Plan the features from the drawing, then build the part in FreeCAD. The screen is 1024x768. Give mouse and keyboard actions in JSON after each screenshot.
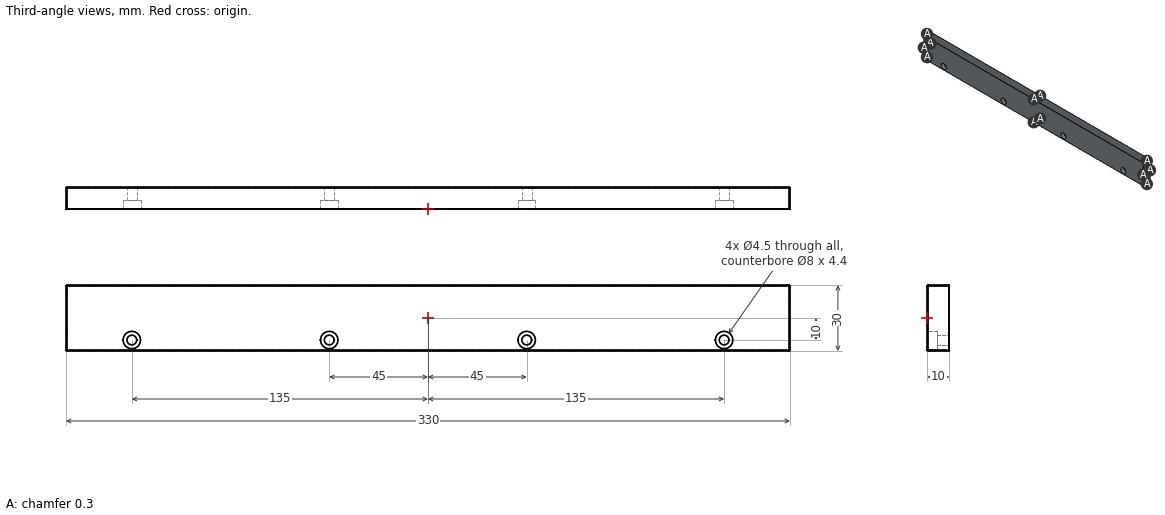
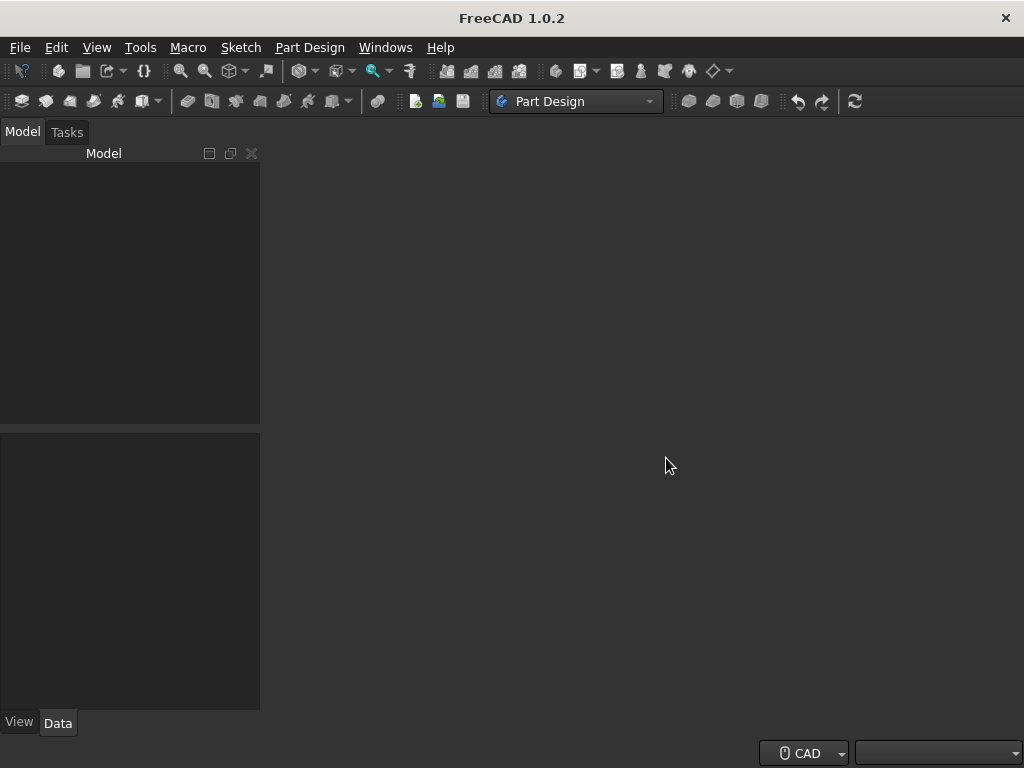
{"action": "left_click", "coordinate": [416, 102]}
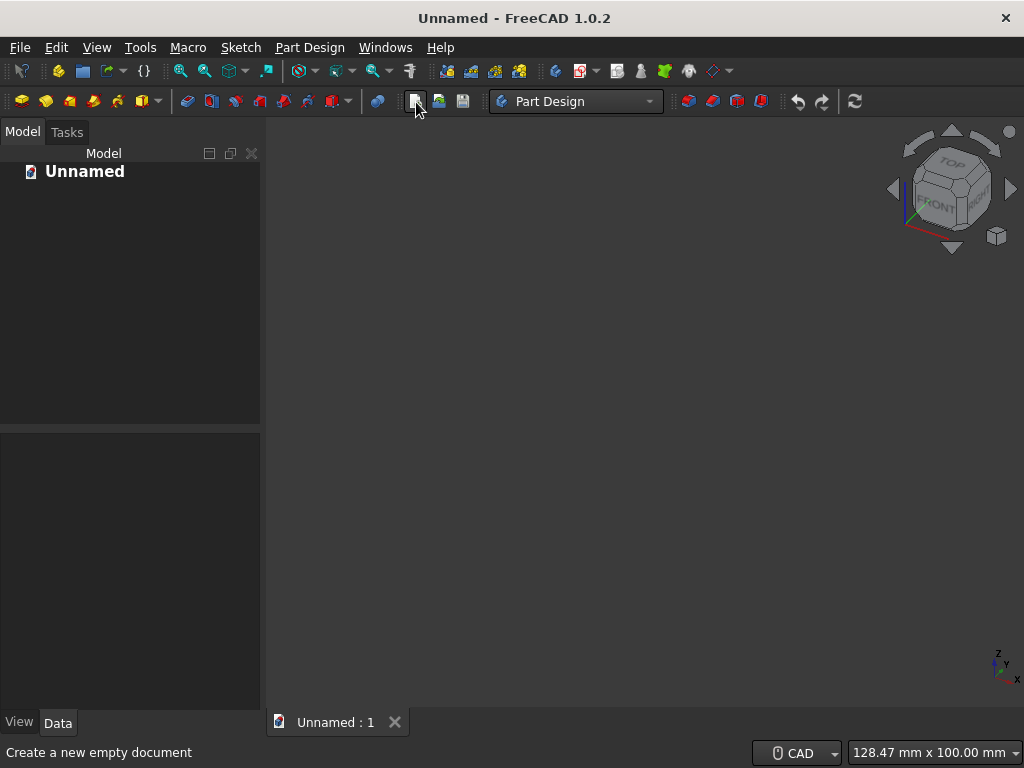
{"action": "left_click", "coordinate": [580, 72]}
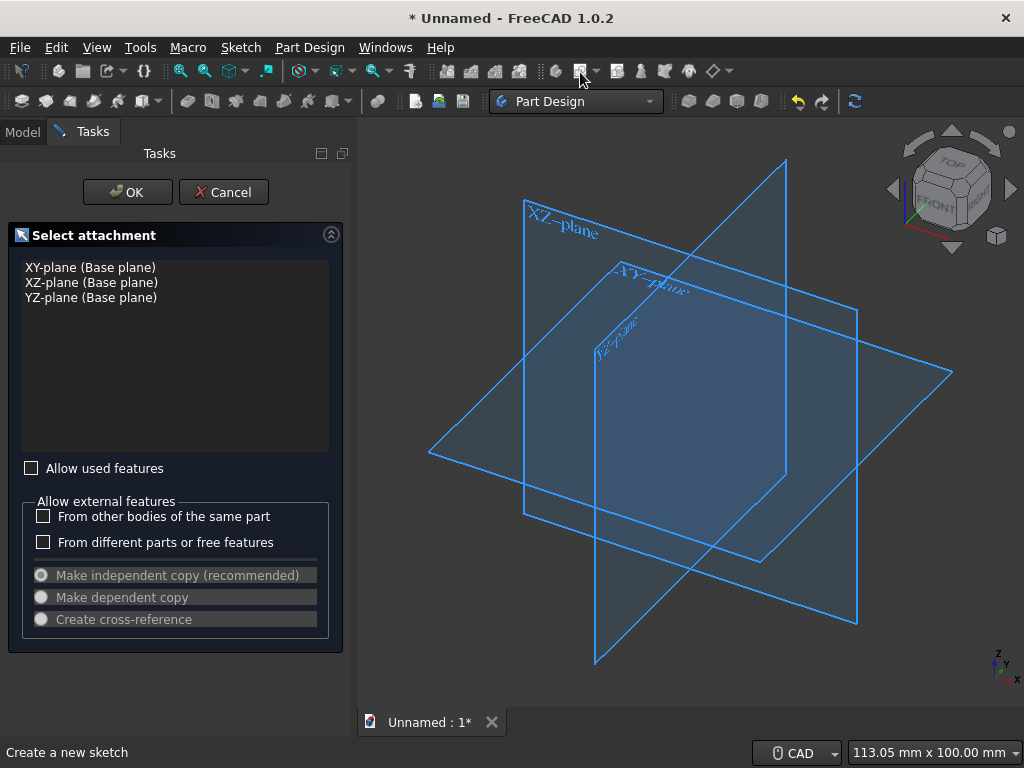
{"action": "left_click", "coordinate": [82, 282]}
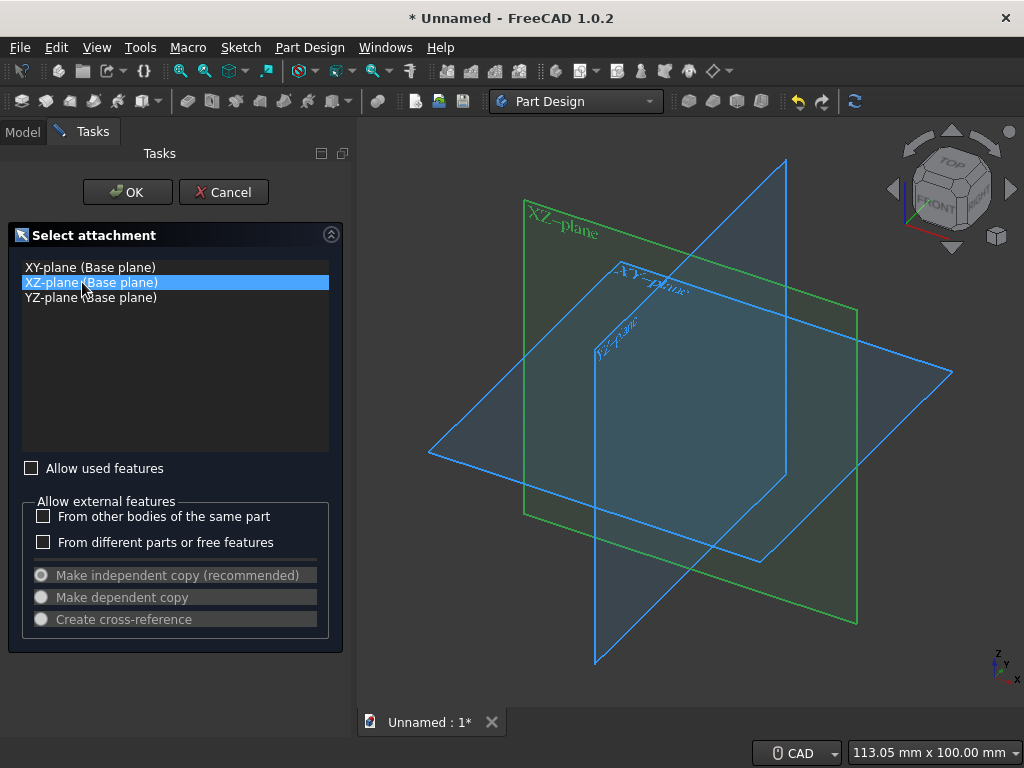
{"action": "left_click", "coordinate": [128, 192]}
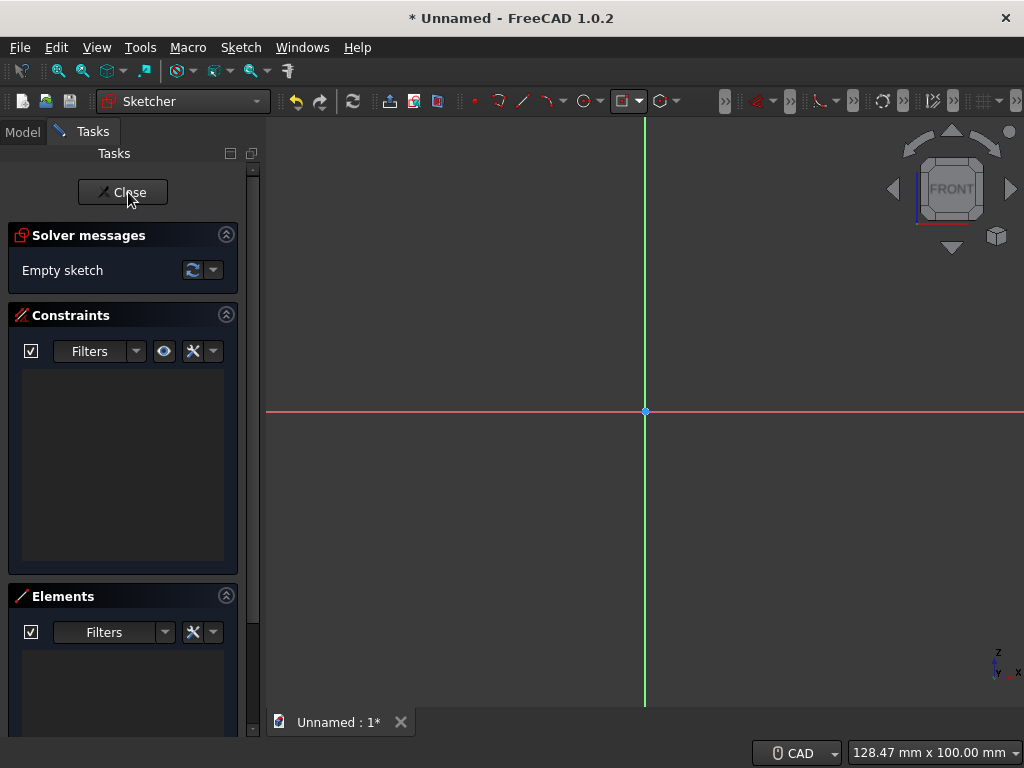
{"action": "scroll", "coordinate": [559, 412], "scroll_direction": "down", "scroll_amount": 8}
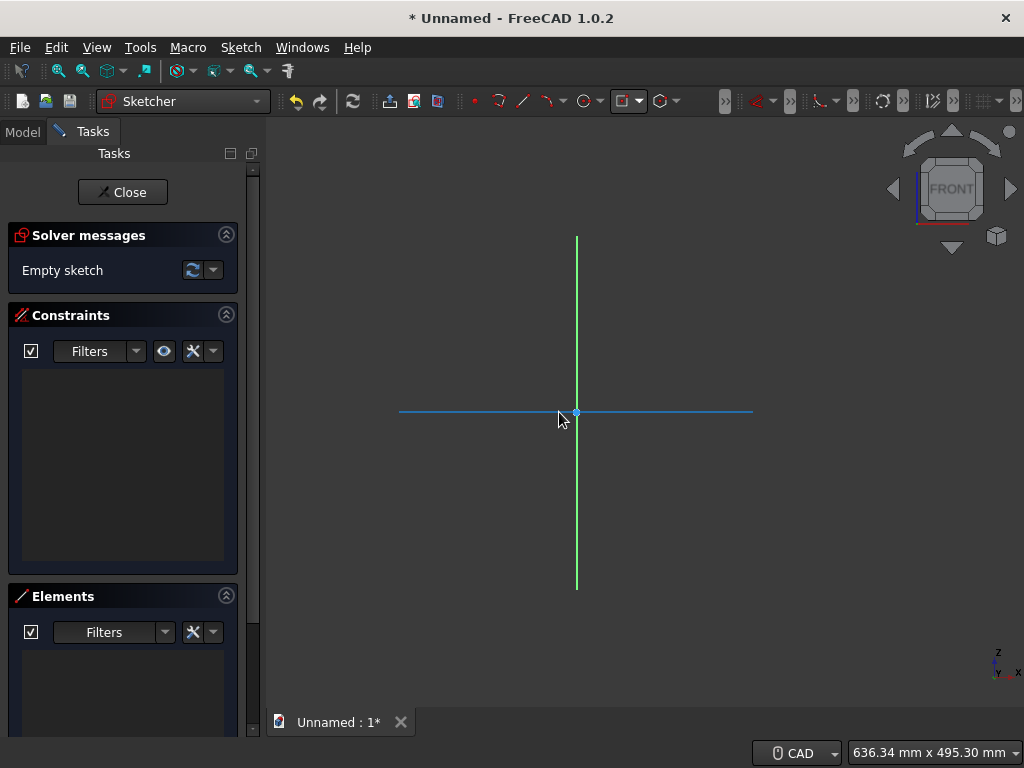
{"action": "left_click", "coordinate": [622, 102]}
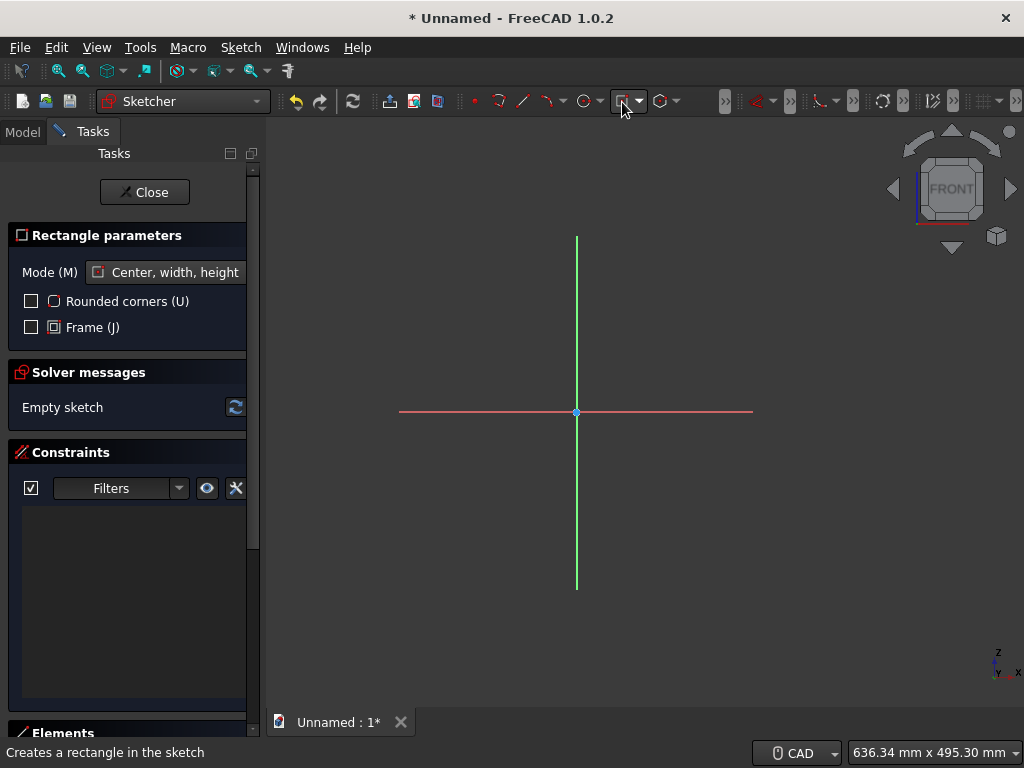
{"action": "left_click", "coordinate": [577, 412]}
{"action": "left_click", "coordinate": [773, 395]}
{"action": "key", "text": "Escape"}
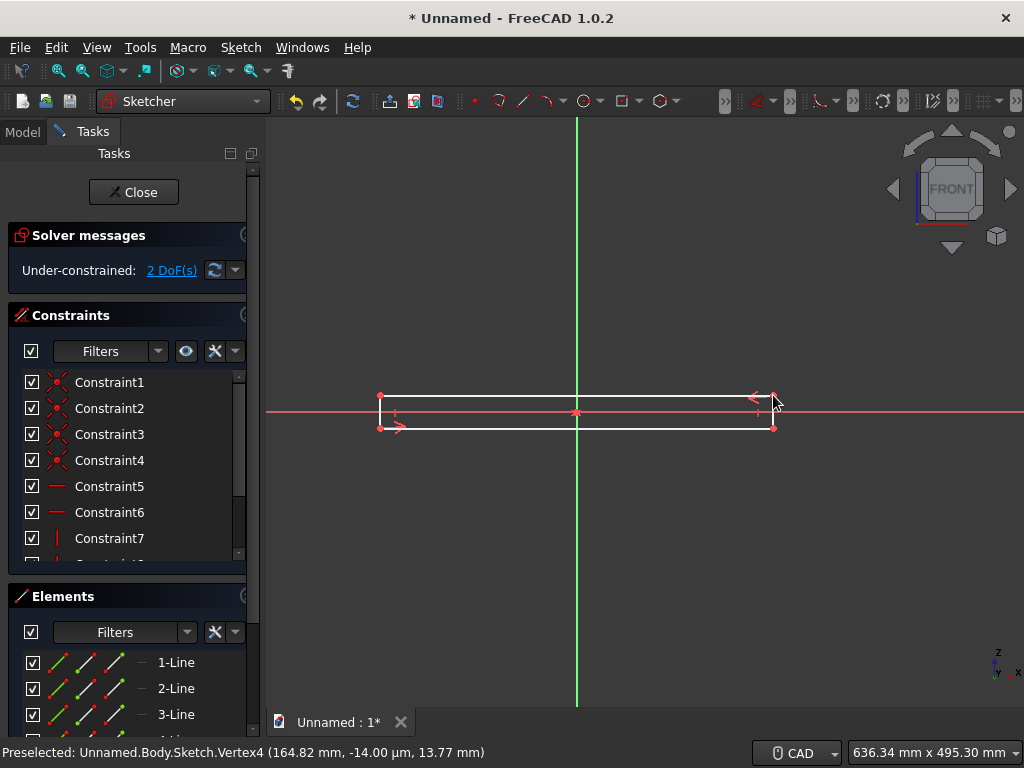
{"action": "left_click", "coordinate": [756, 102]}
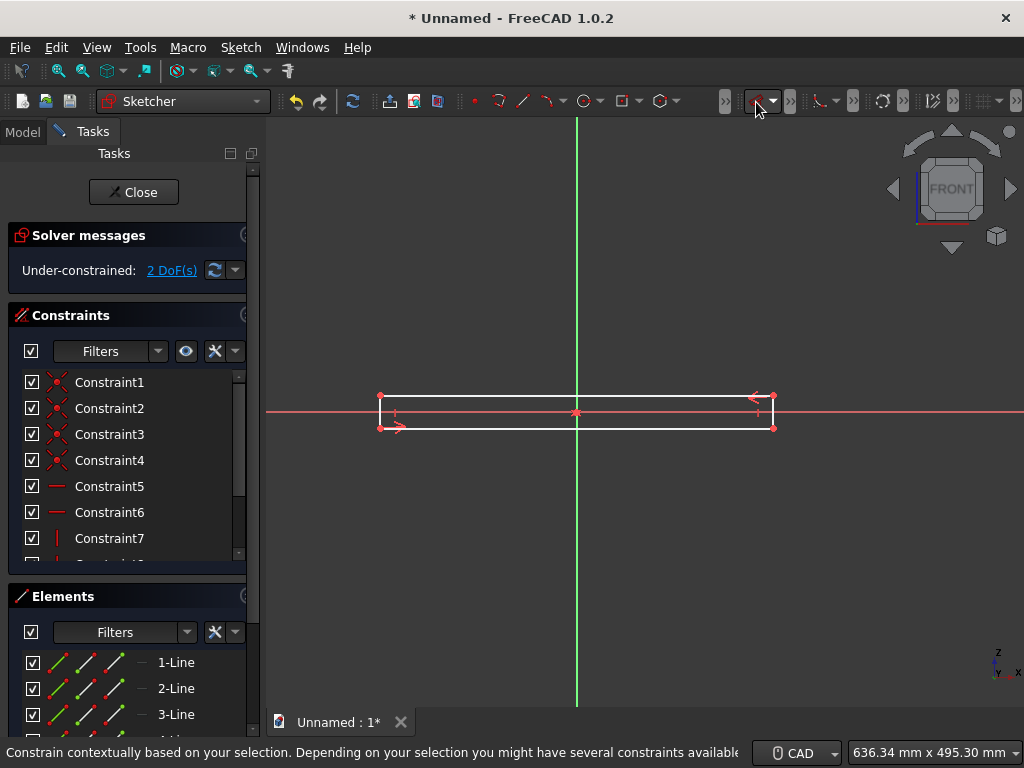
{"action": "left_click", "coordinate": [773, 416]}
{"action": "left_click", "coordinate": [807, 405]}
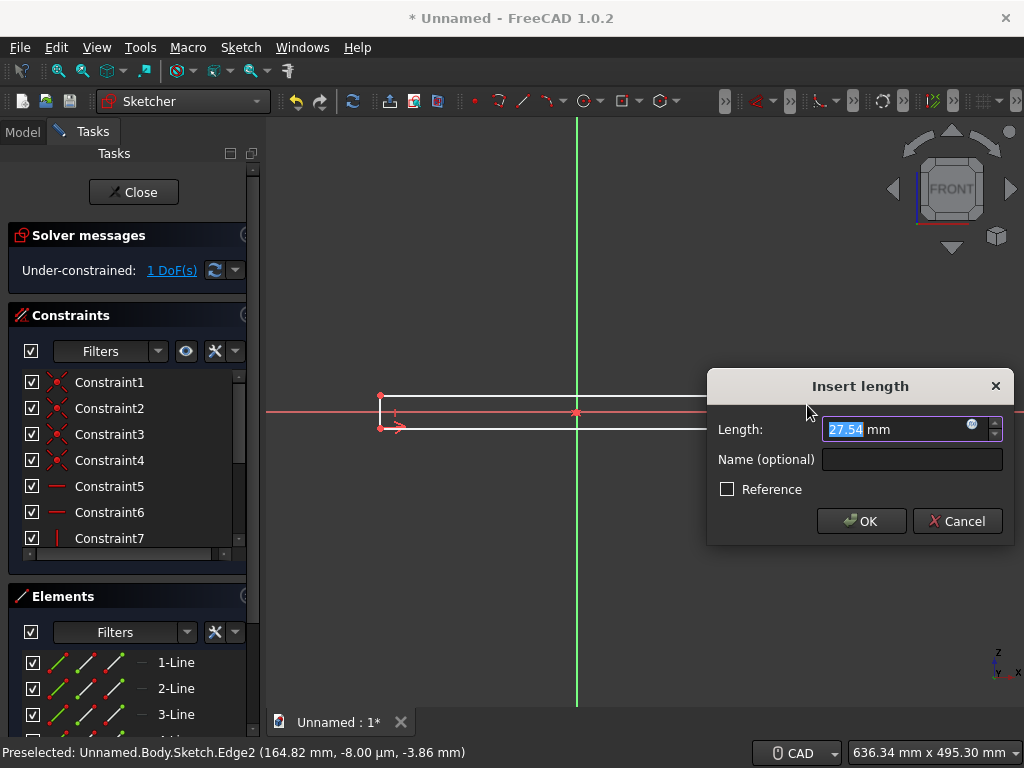
{"action": "type", "text": "30"}
{"action": "key", "text": "Return"}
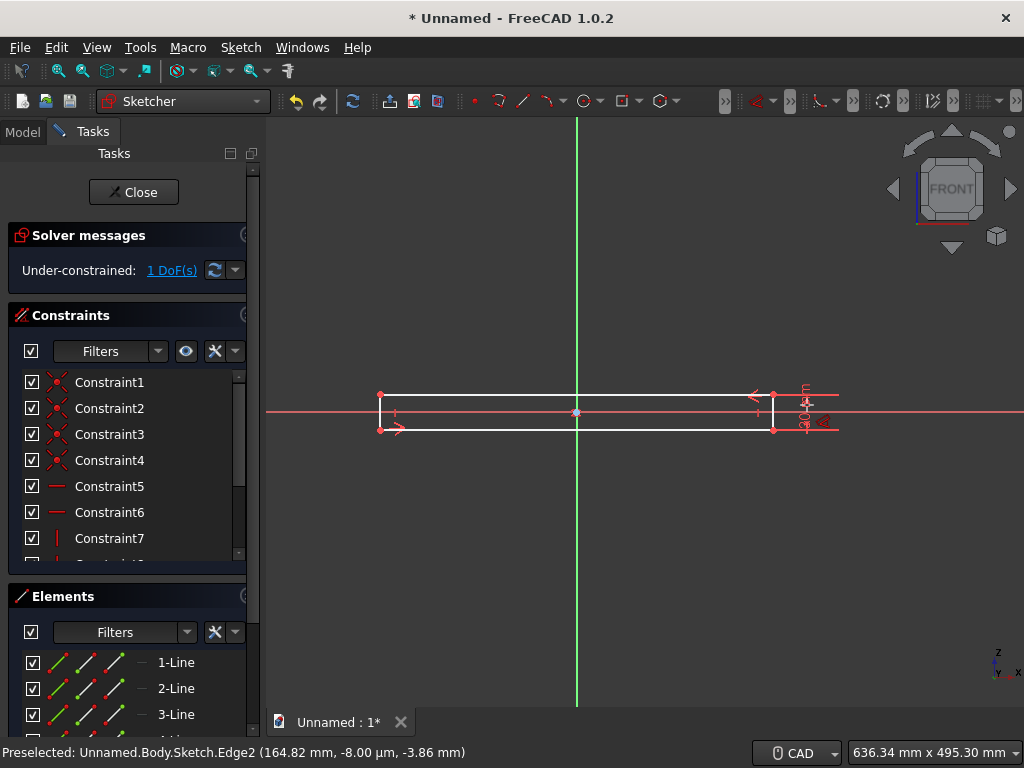
{"action": "left_click", "coordinate": [498, 430]}
{"action": "left_click", "coordinate": [486, 464]}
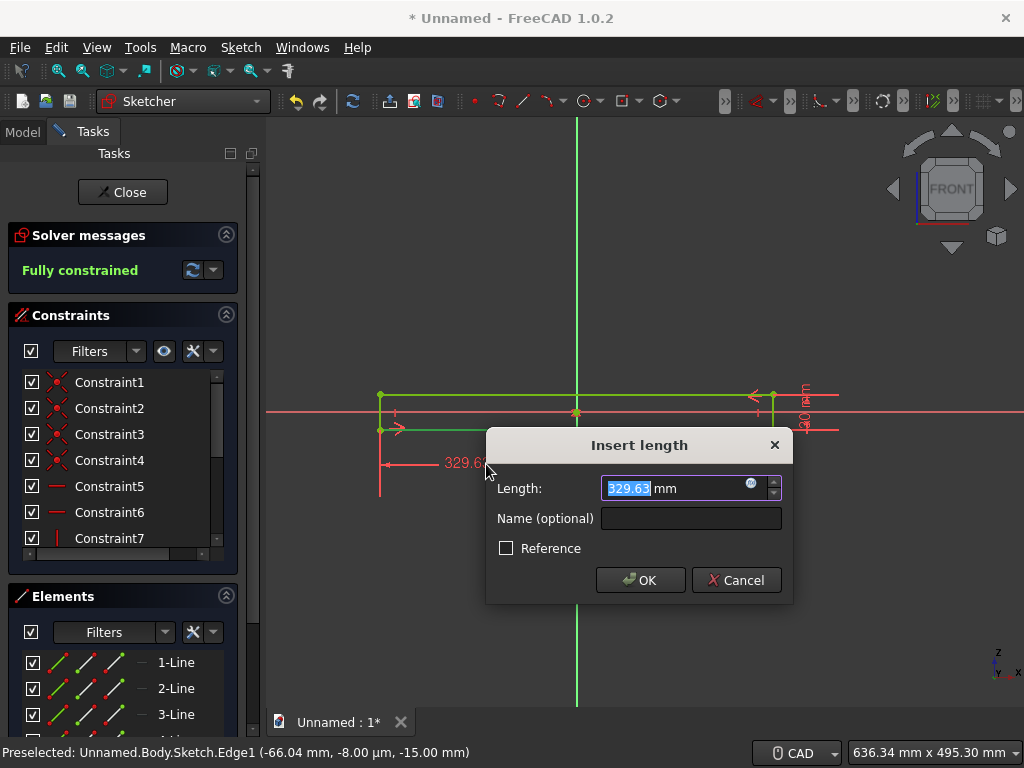
{"action": "type", "text": "330"}
{"action": "key", "text": "Return"}
{"action": "key", "text": "Escape"}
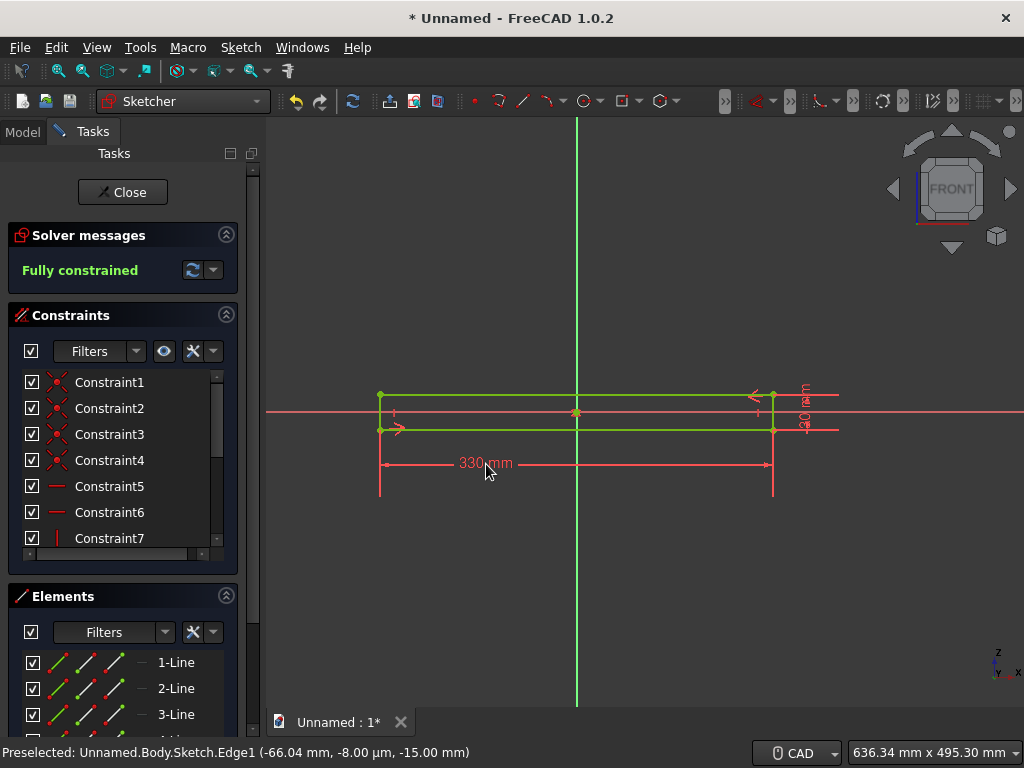
{"action": "left_click", "coordinate": [123, 192]}